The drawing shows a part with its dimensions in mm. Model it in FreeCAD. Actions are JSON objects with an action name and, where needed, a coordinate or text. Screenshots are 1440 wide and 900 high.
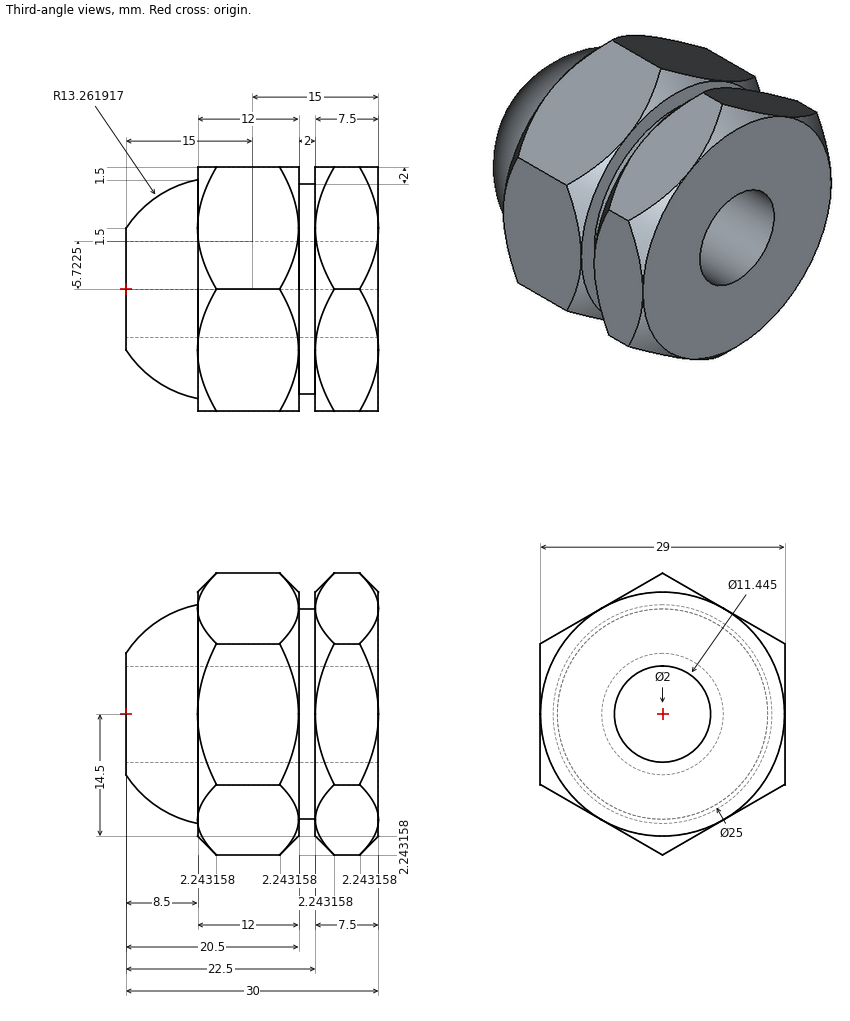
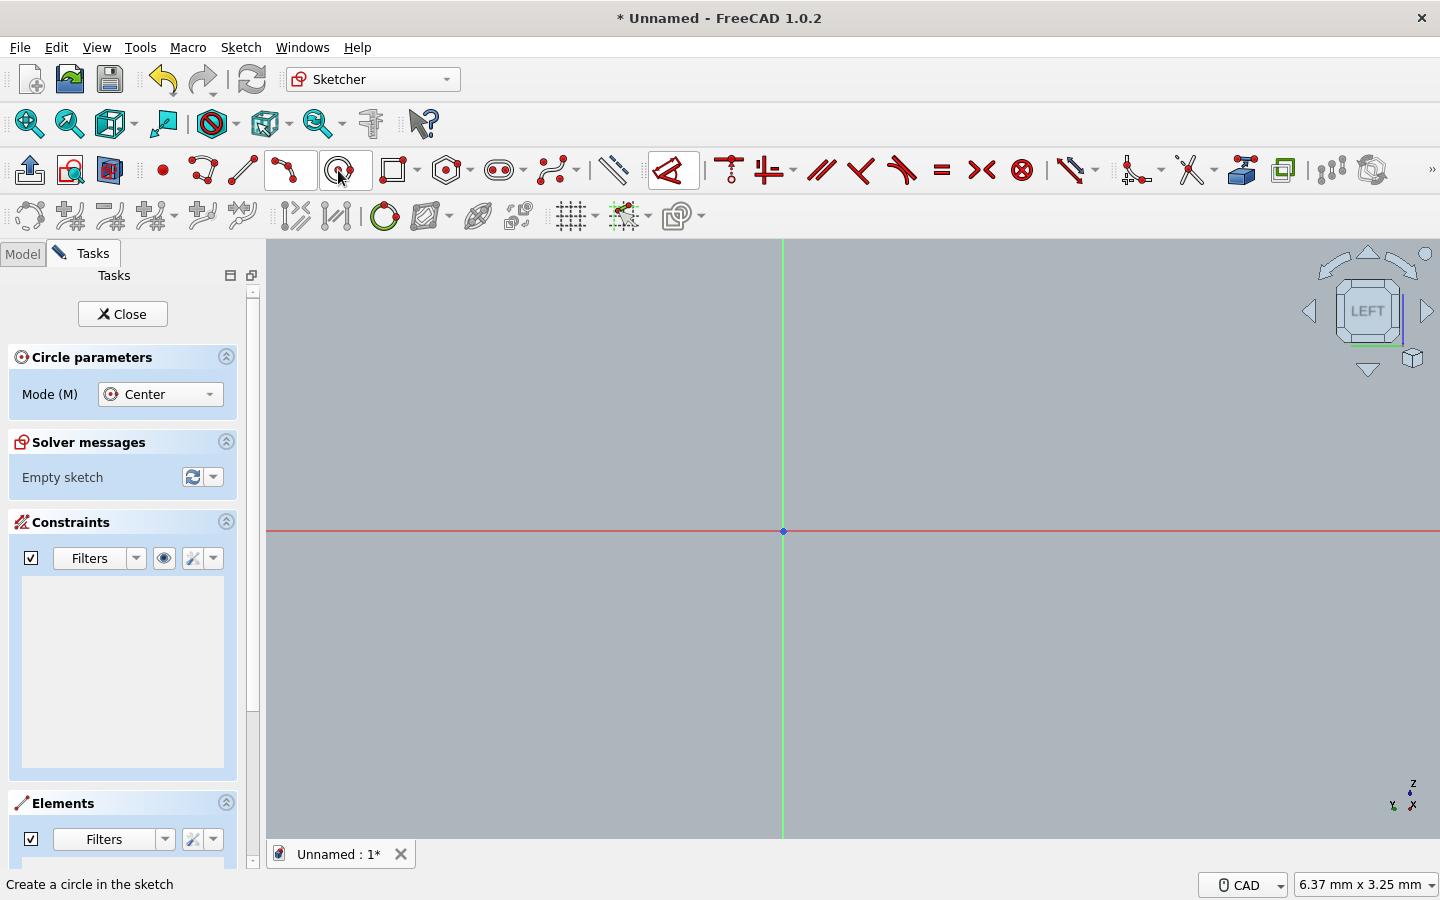
{"action": "left_click", "coordinate": [783, 531]}
{"action": "left_click", "coordinate": [914, 401]}
{"action": "key", "text": "Escape"}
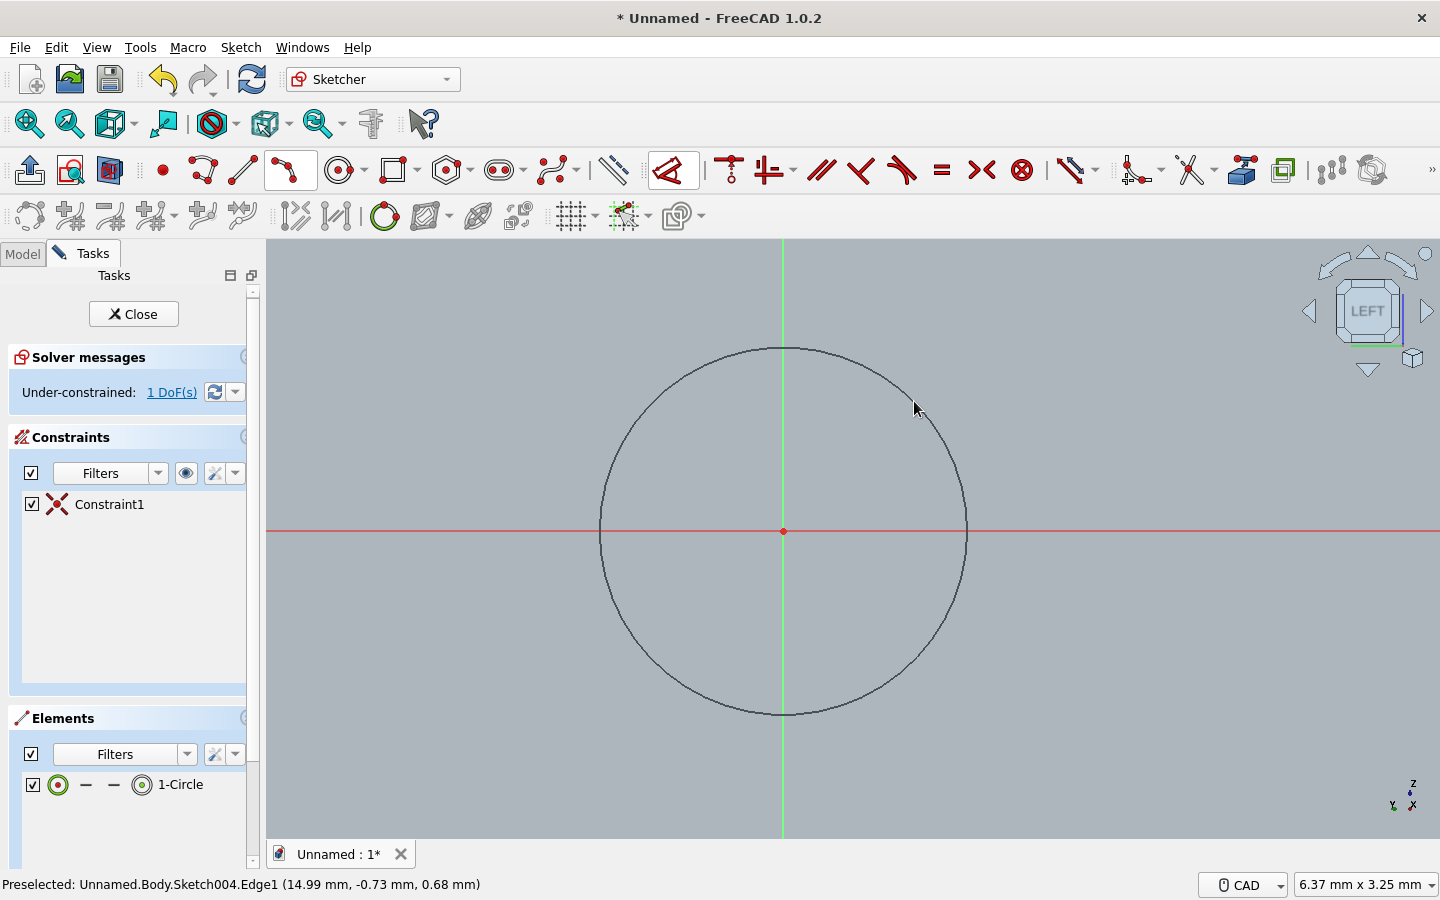
{"action": "left_click", "coordinate": [913, 401]}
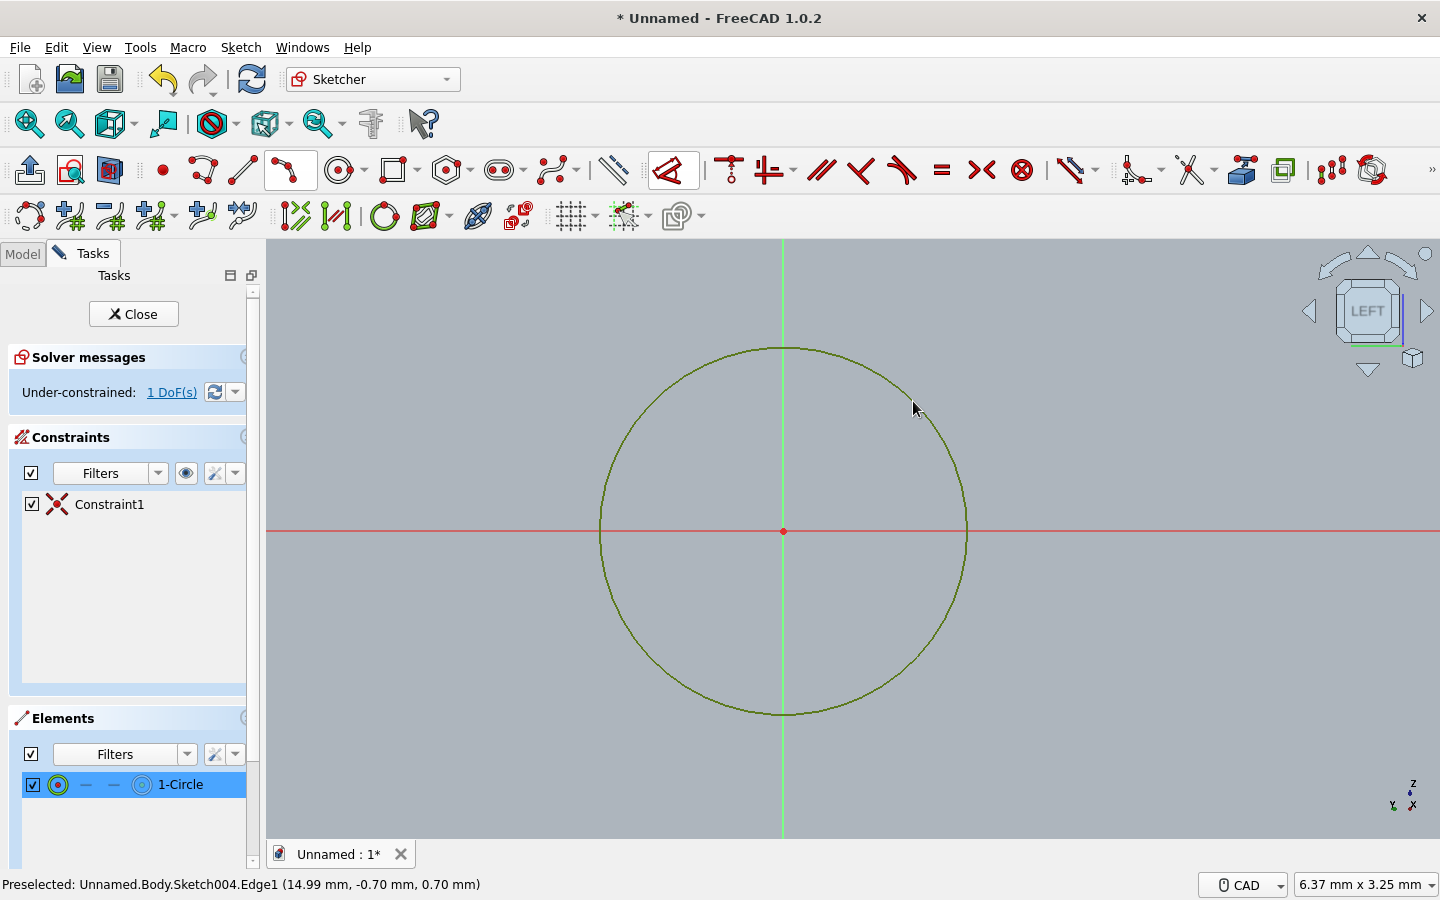
{"action": "left_click", "coordinate": [694, 170]}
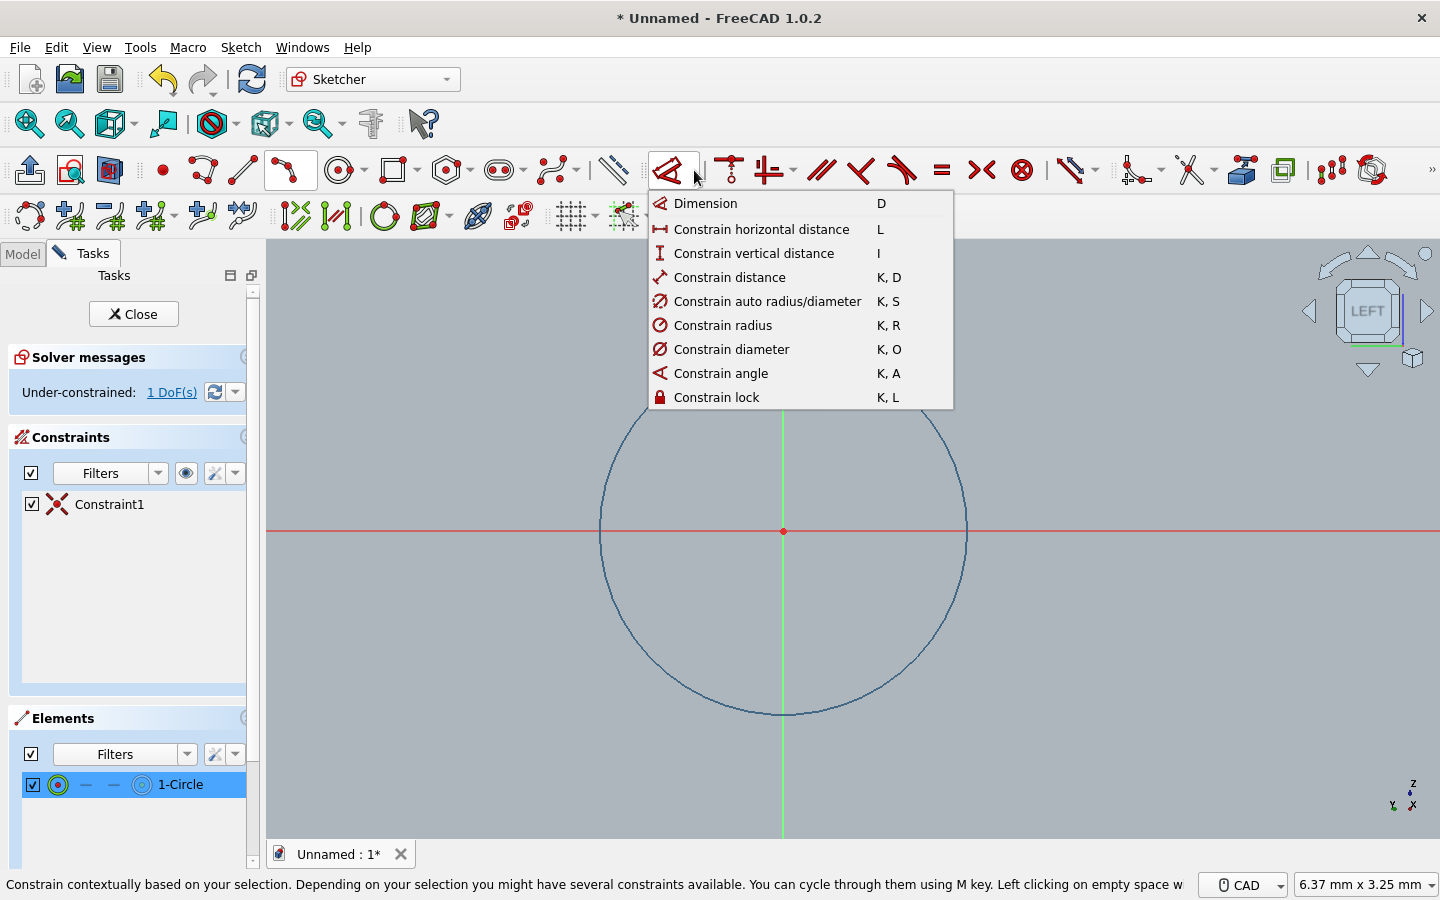
{"action": "left_click", "coordinate": [801, 349]}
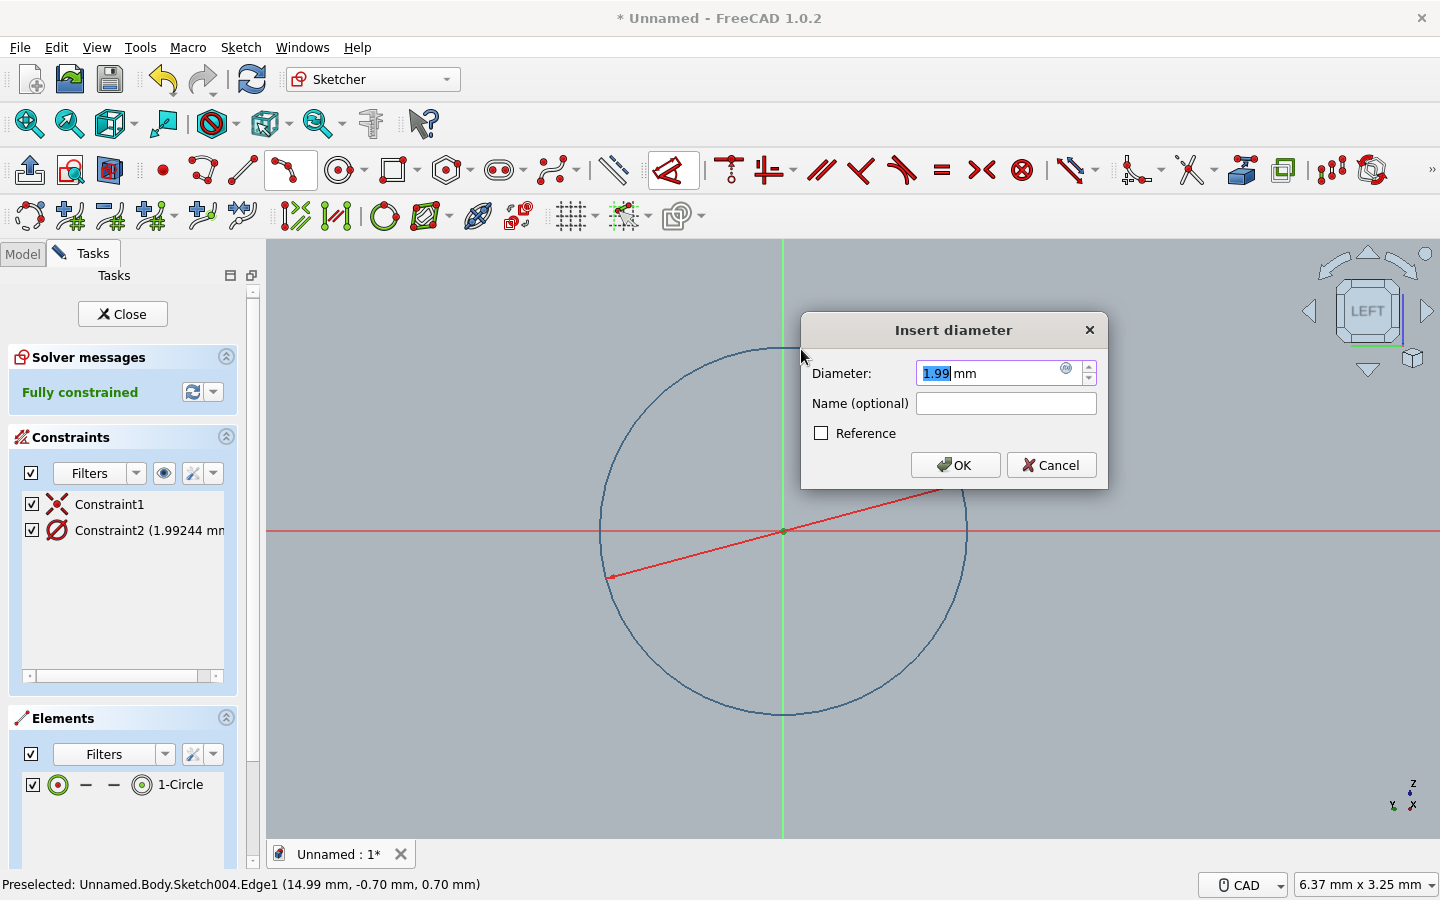
{"action": "type", "text": "2"}
{"action": "key", "text": "Return"}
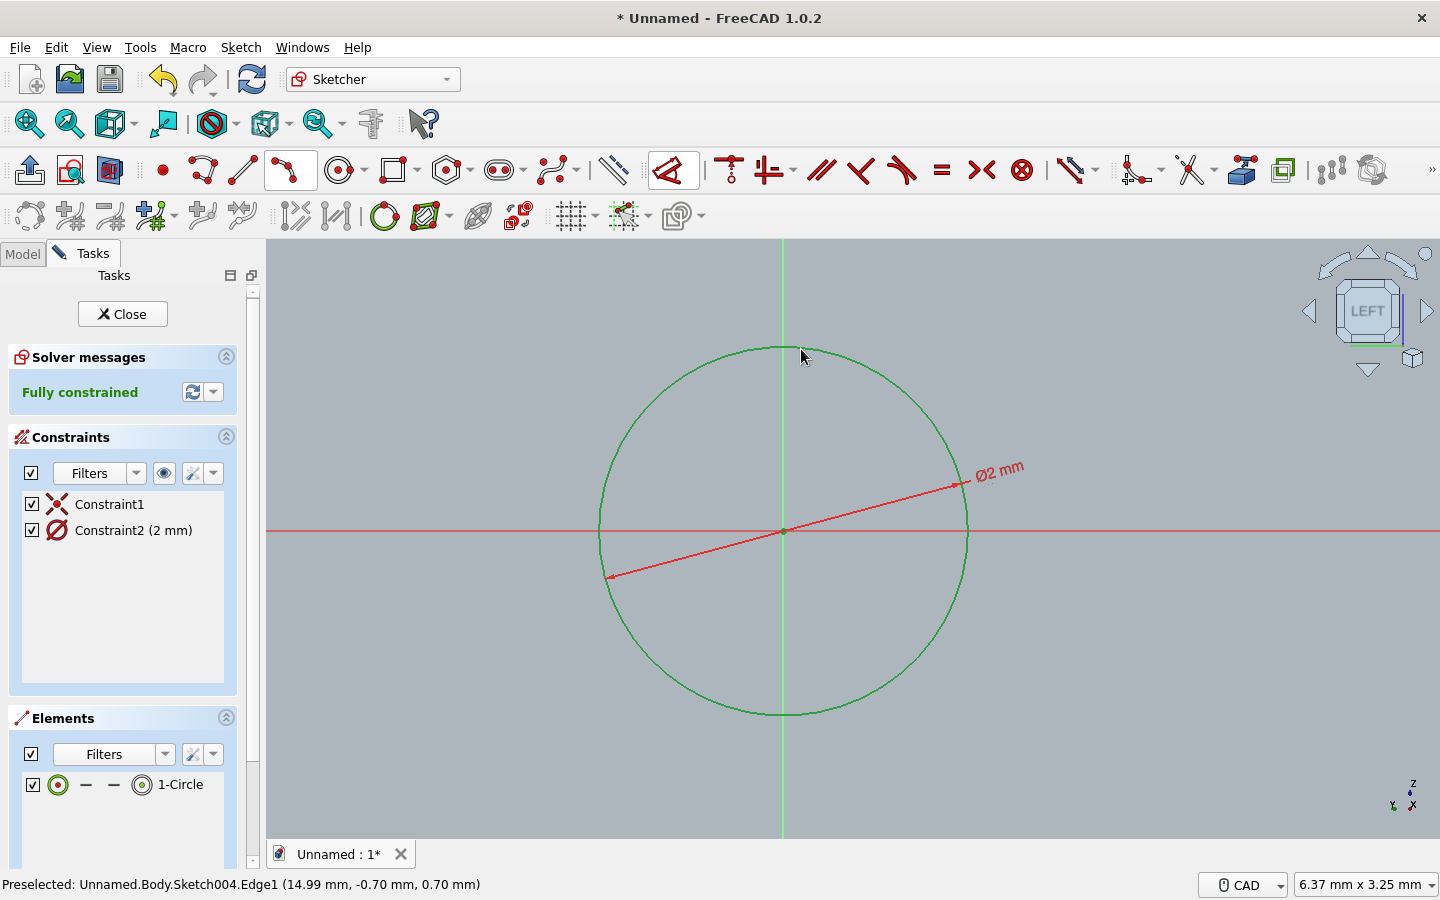
{"action": "left_click", "coordinate": [123, 314]}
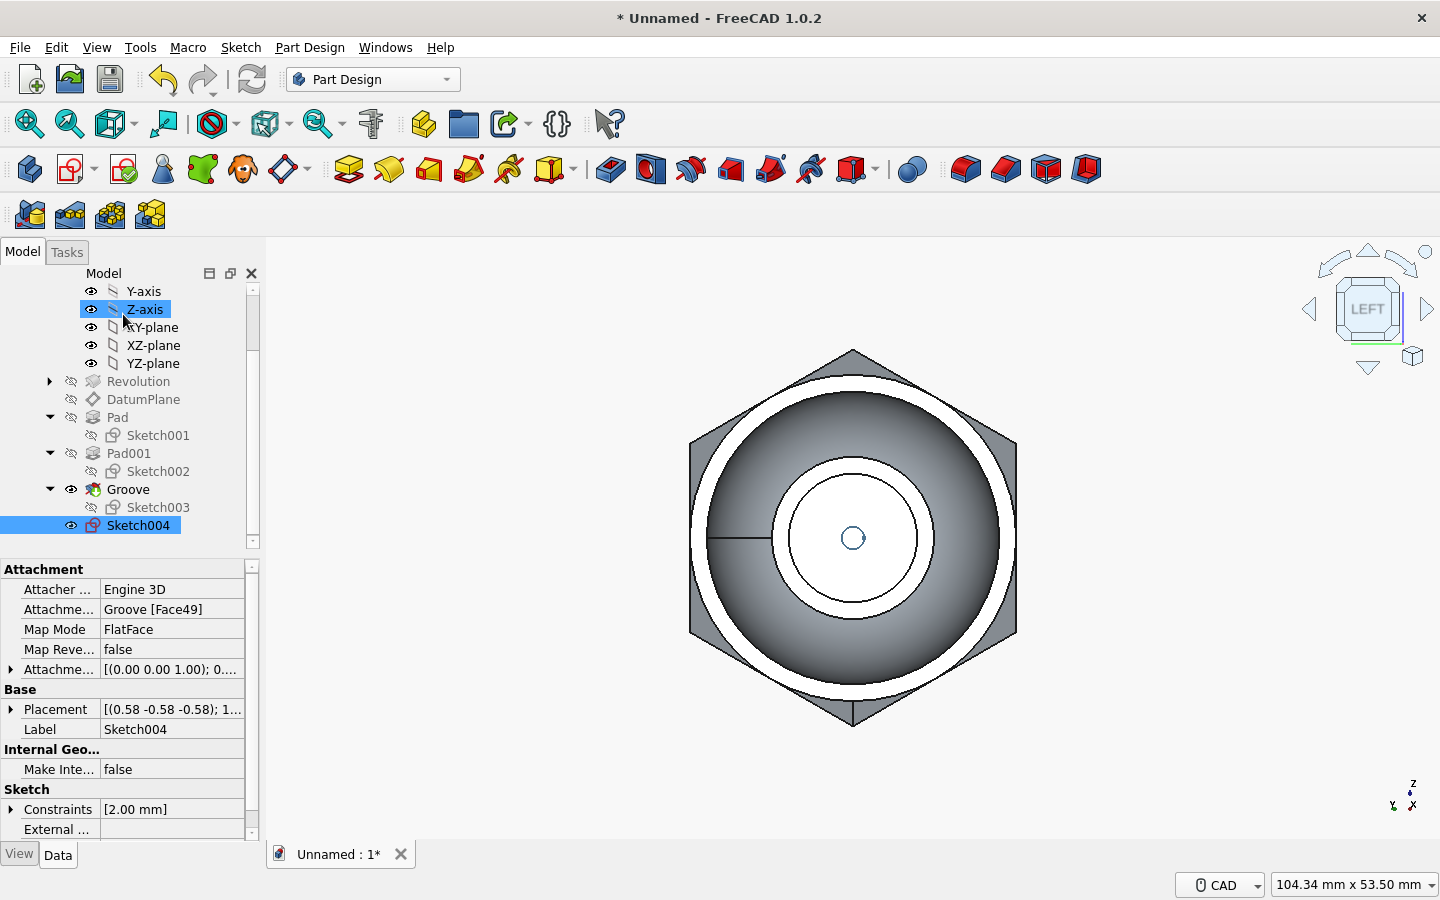
{"action": "left_click", "coordinate": [612, 170]}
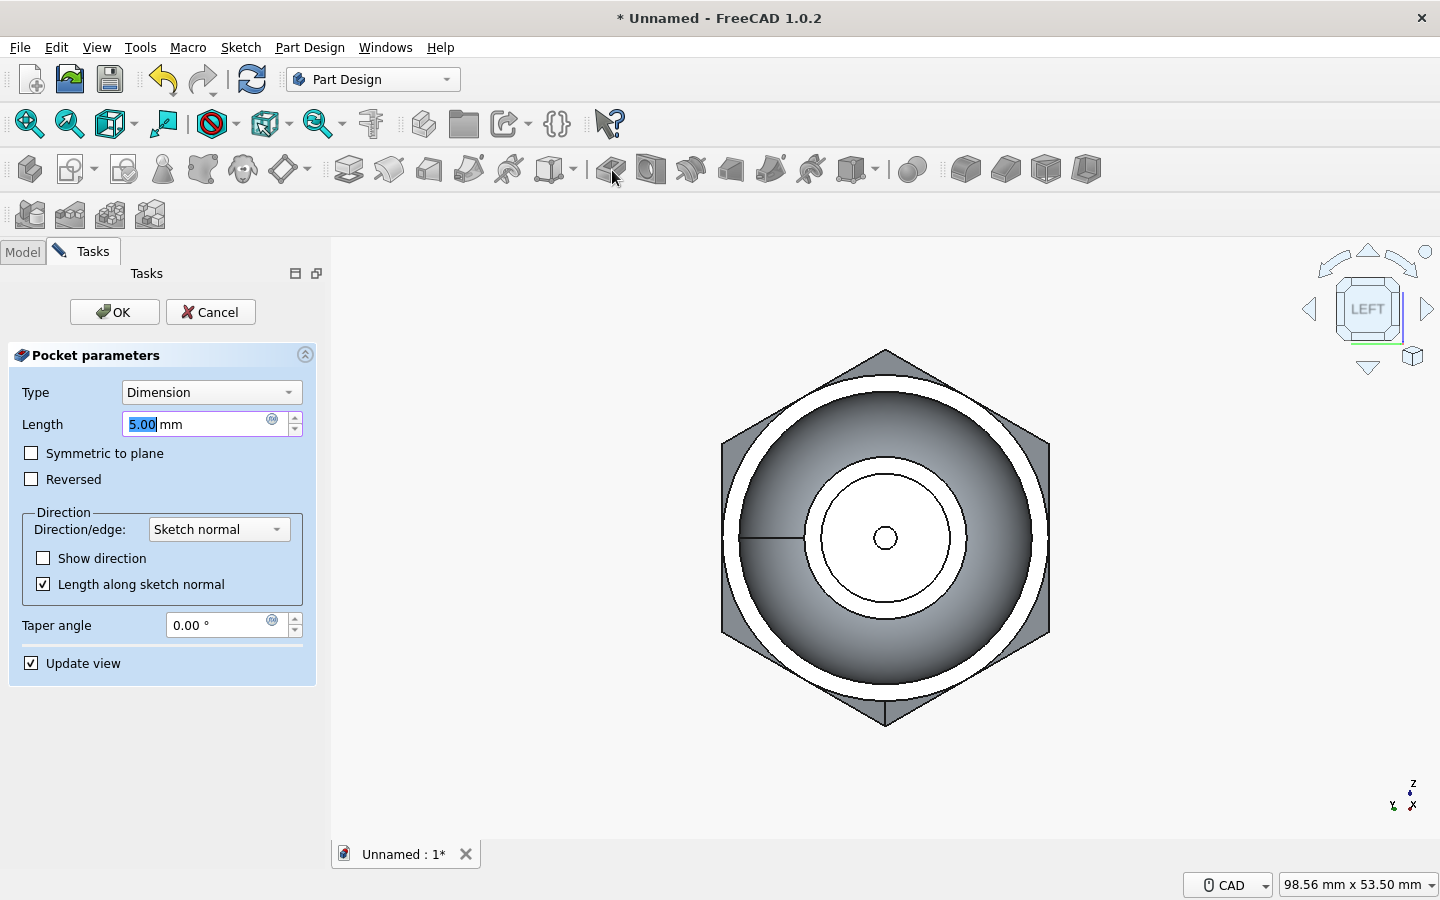
{"action": "left_click", "coordinate": [212, 392]}